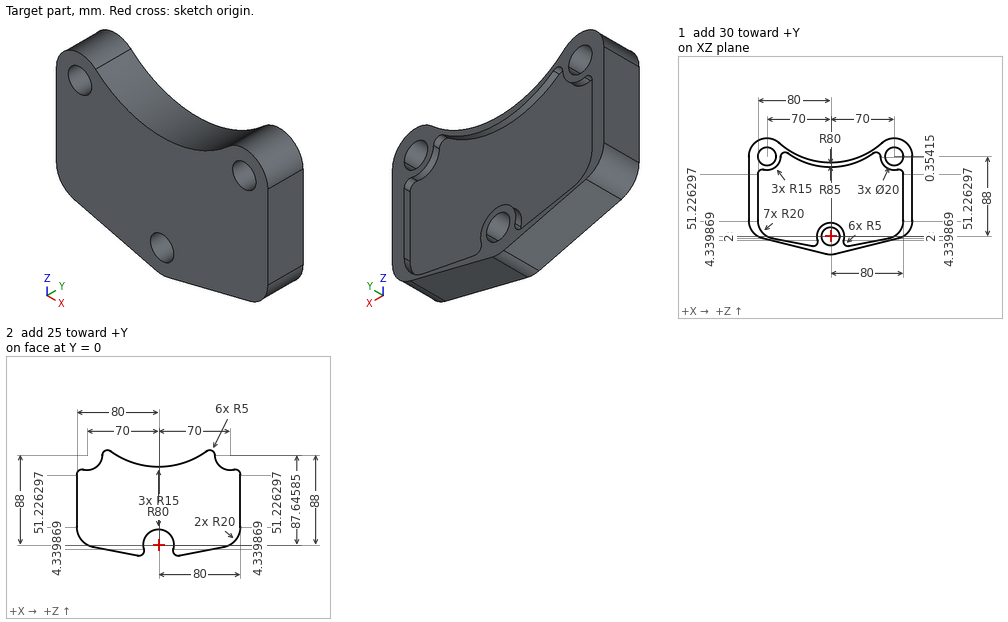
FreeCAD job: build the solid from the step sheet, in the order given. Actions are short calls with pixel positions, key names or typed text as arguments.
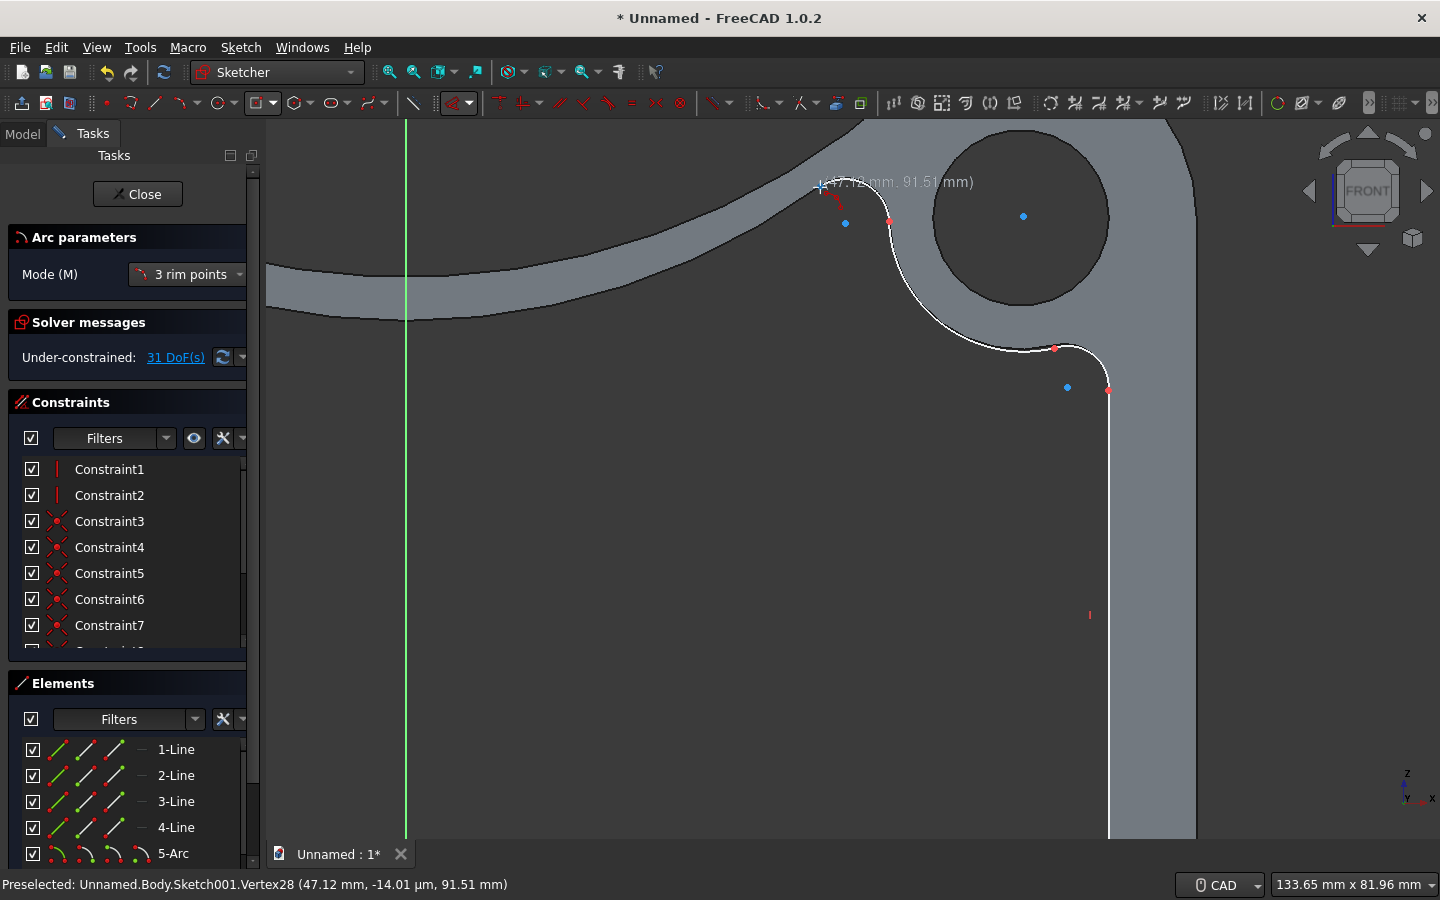
scroll(1093, 353, down, 4)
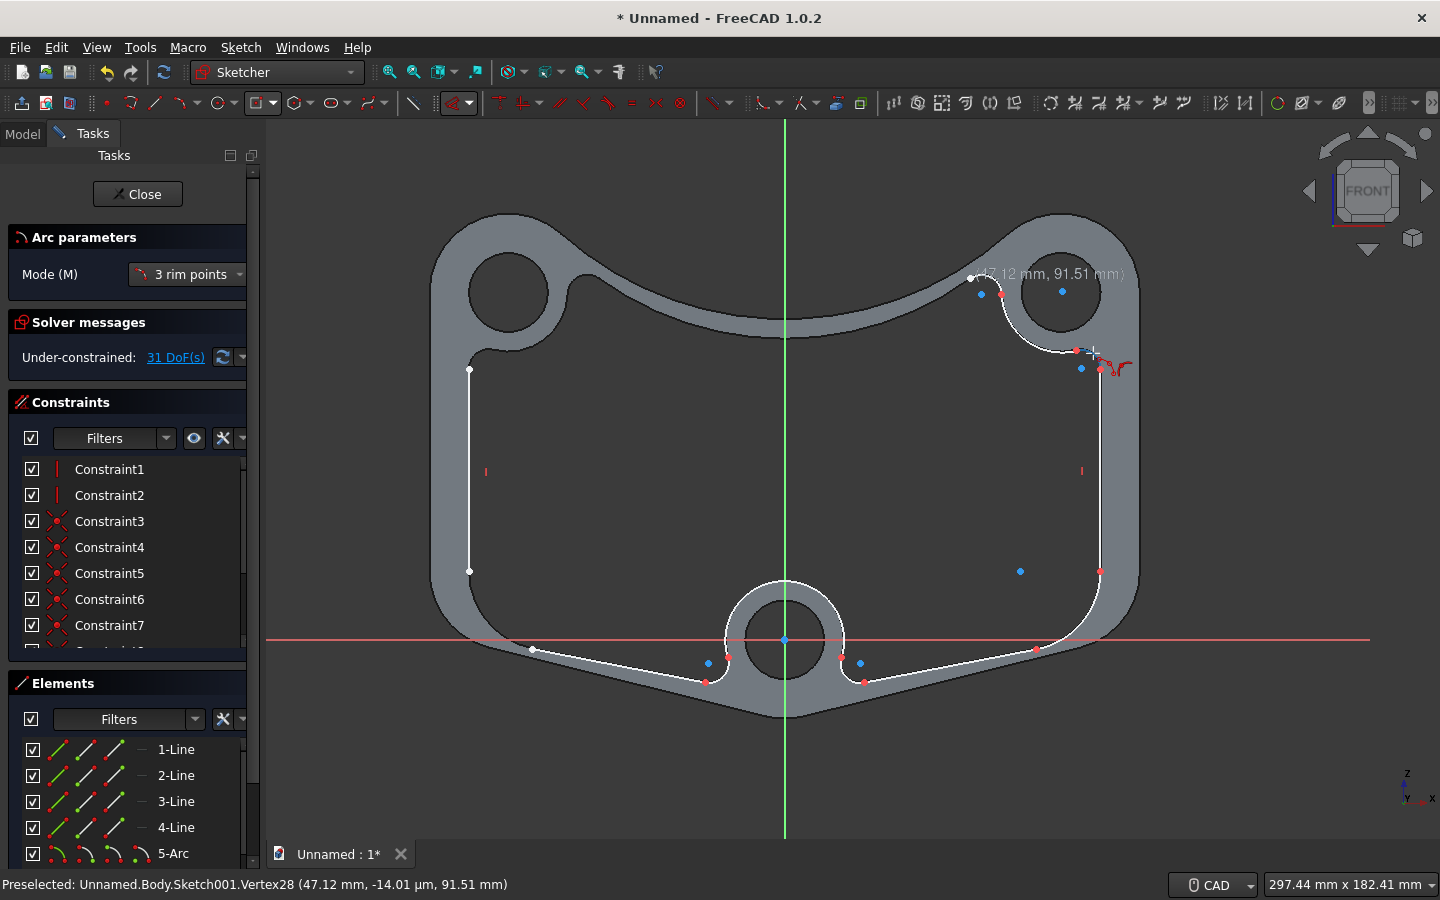
click(599, 278)
click(745, 336)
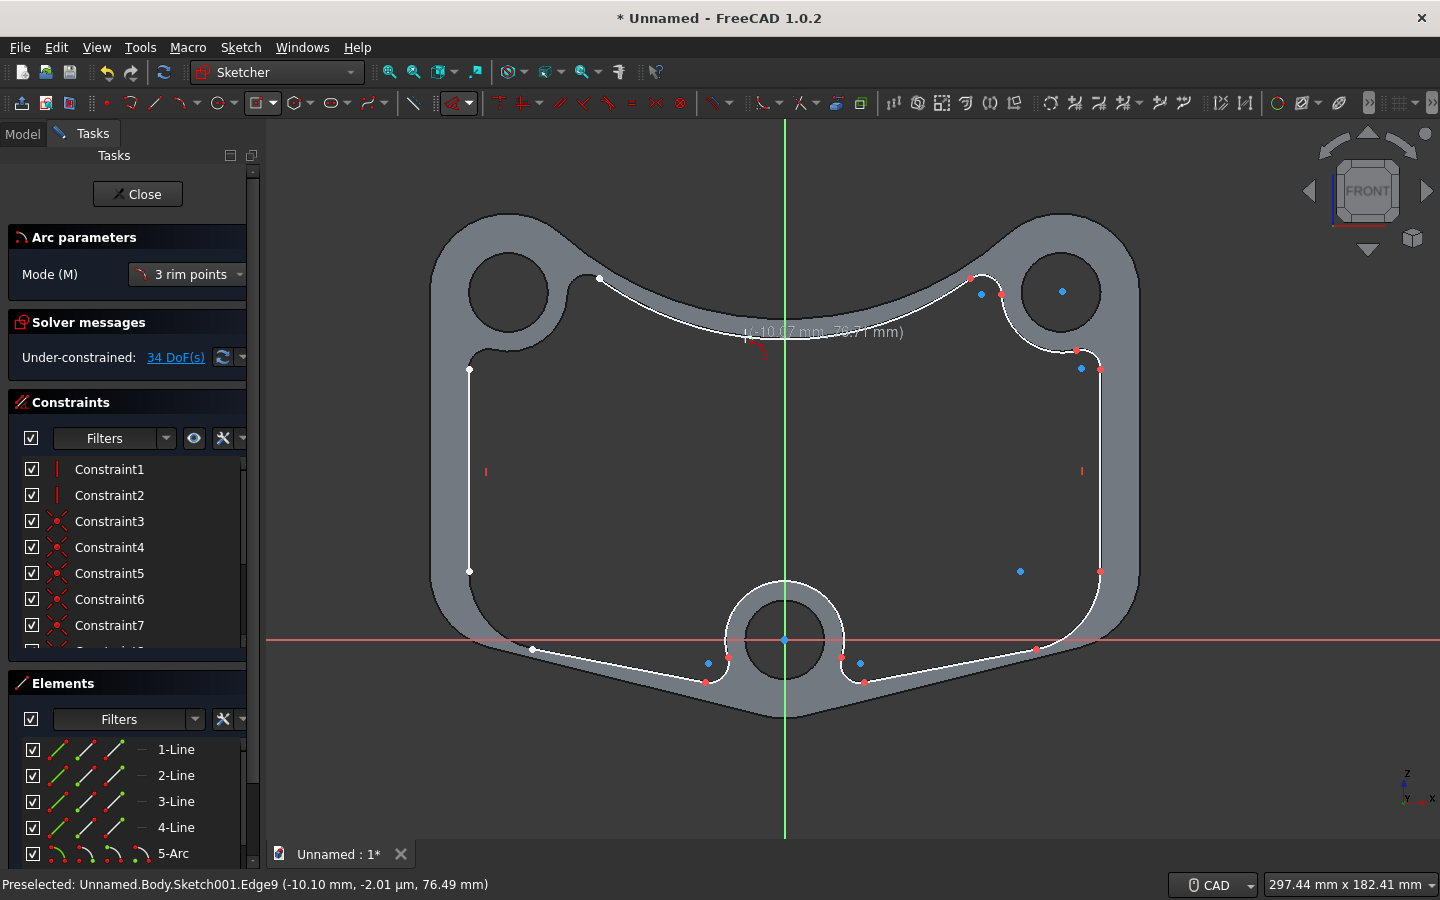
click(599, 279)
click(568, 294)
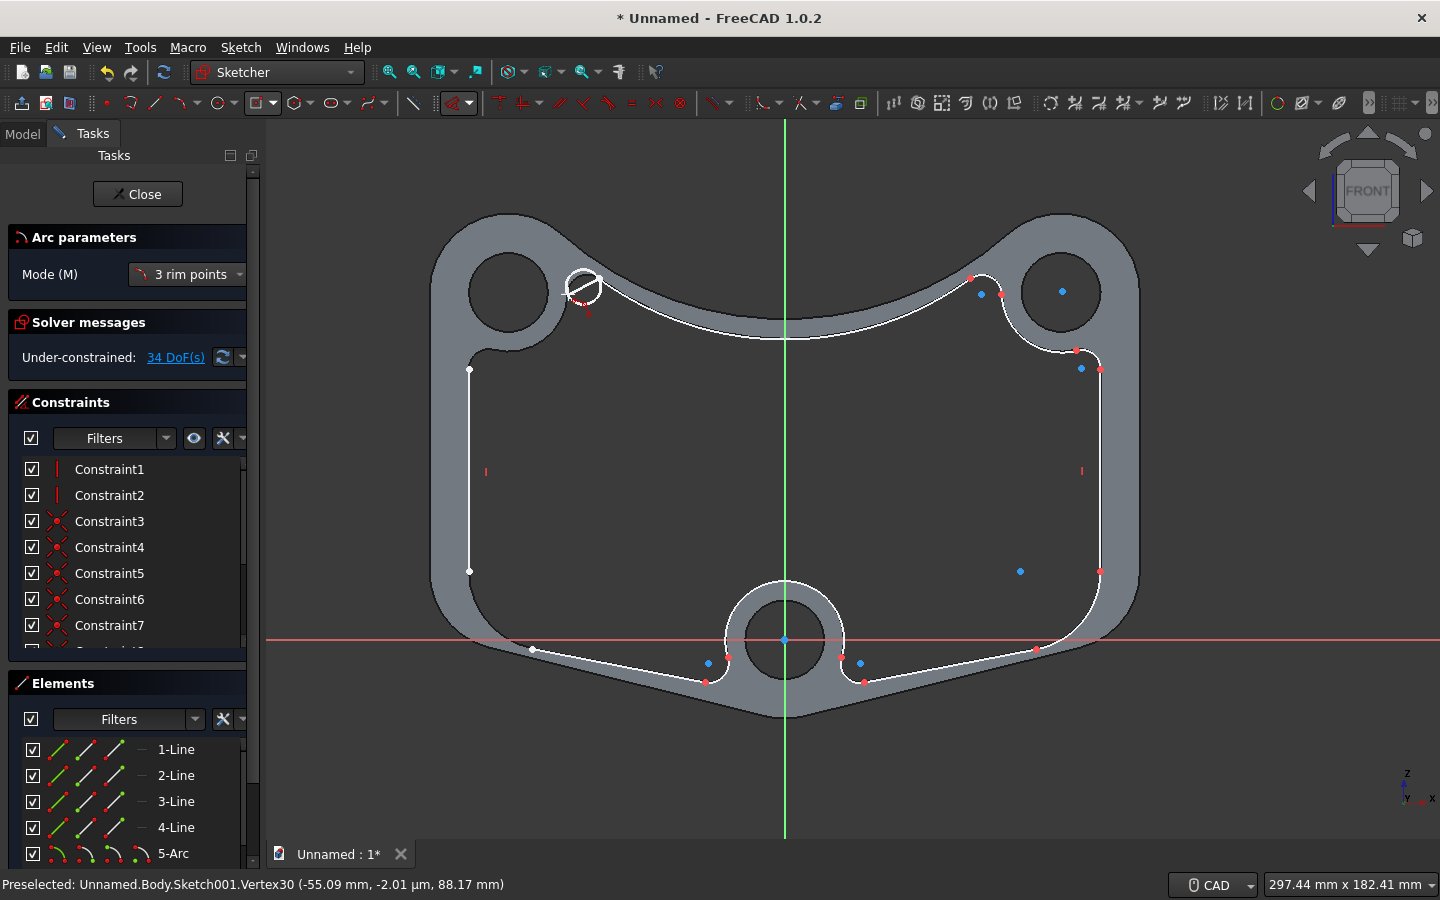
scroll(579, 277, up, 3)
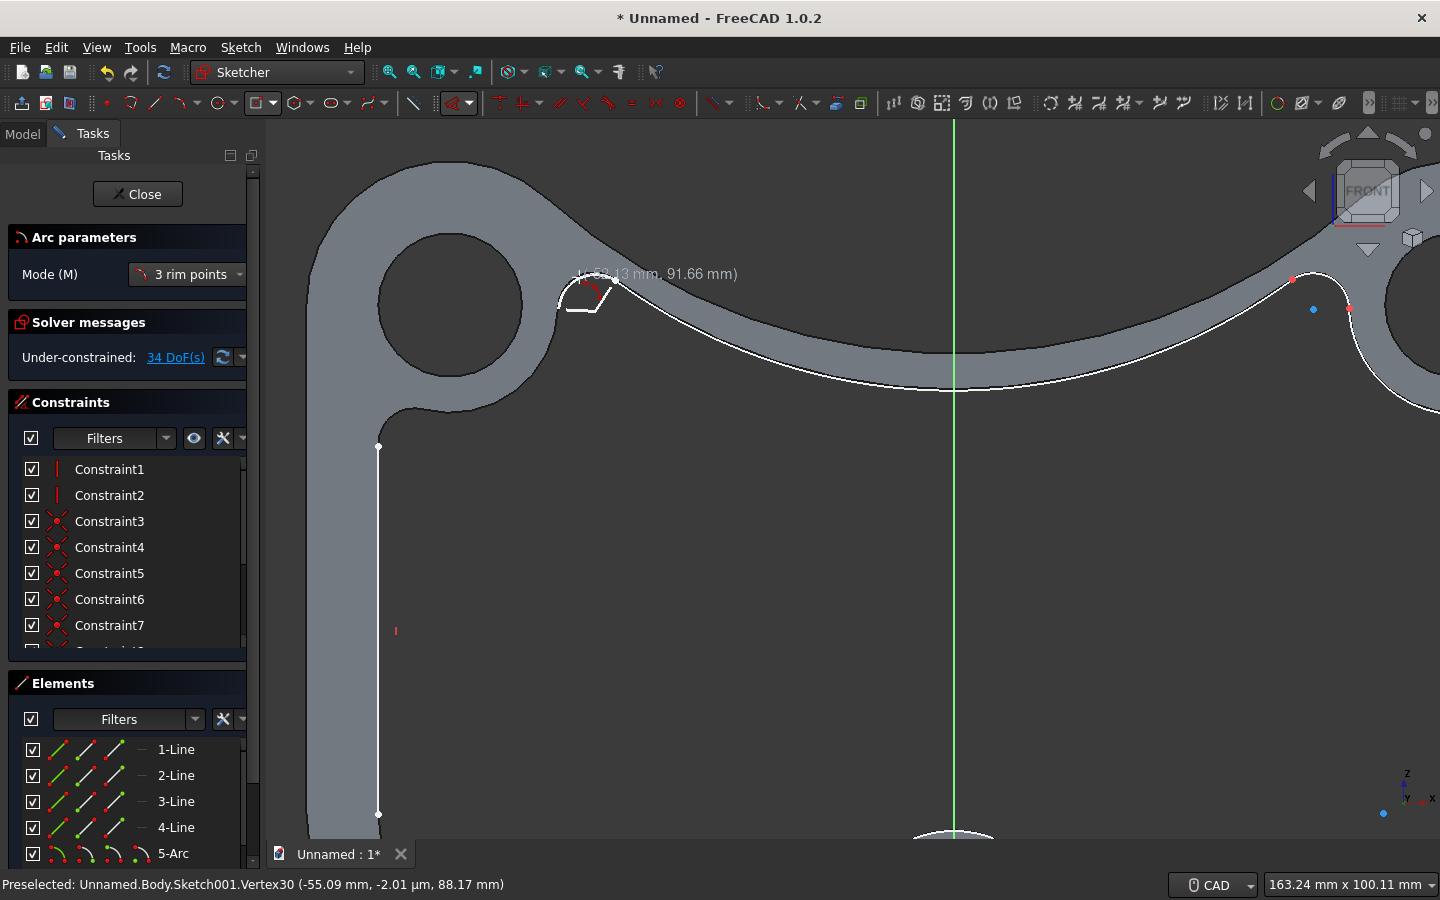
click(578, 276)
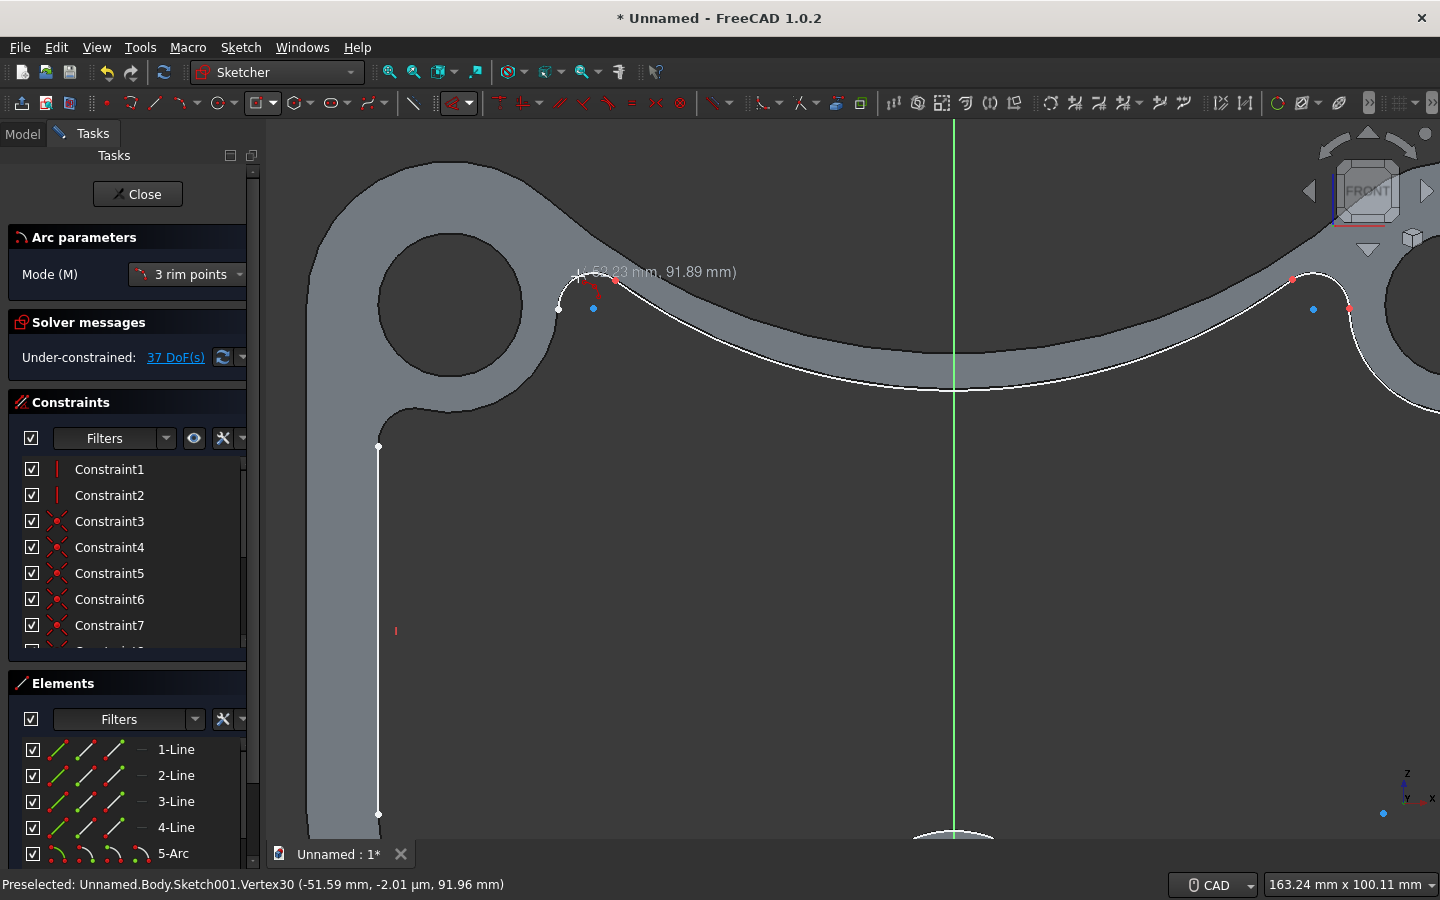
click(559, 310)
click(423, 409)
click(515, 391)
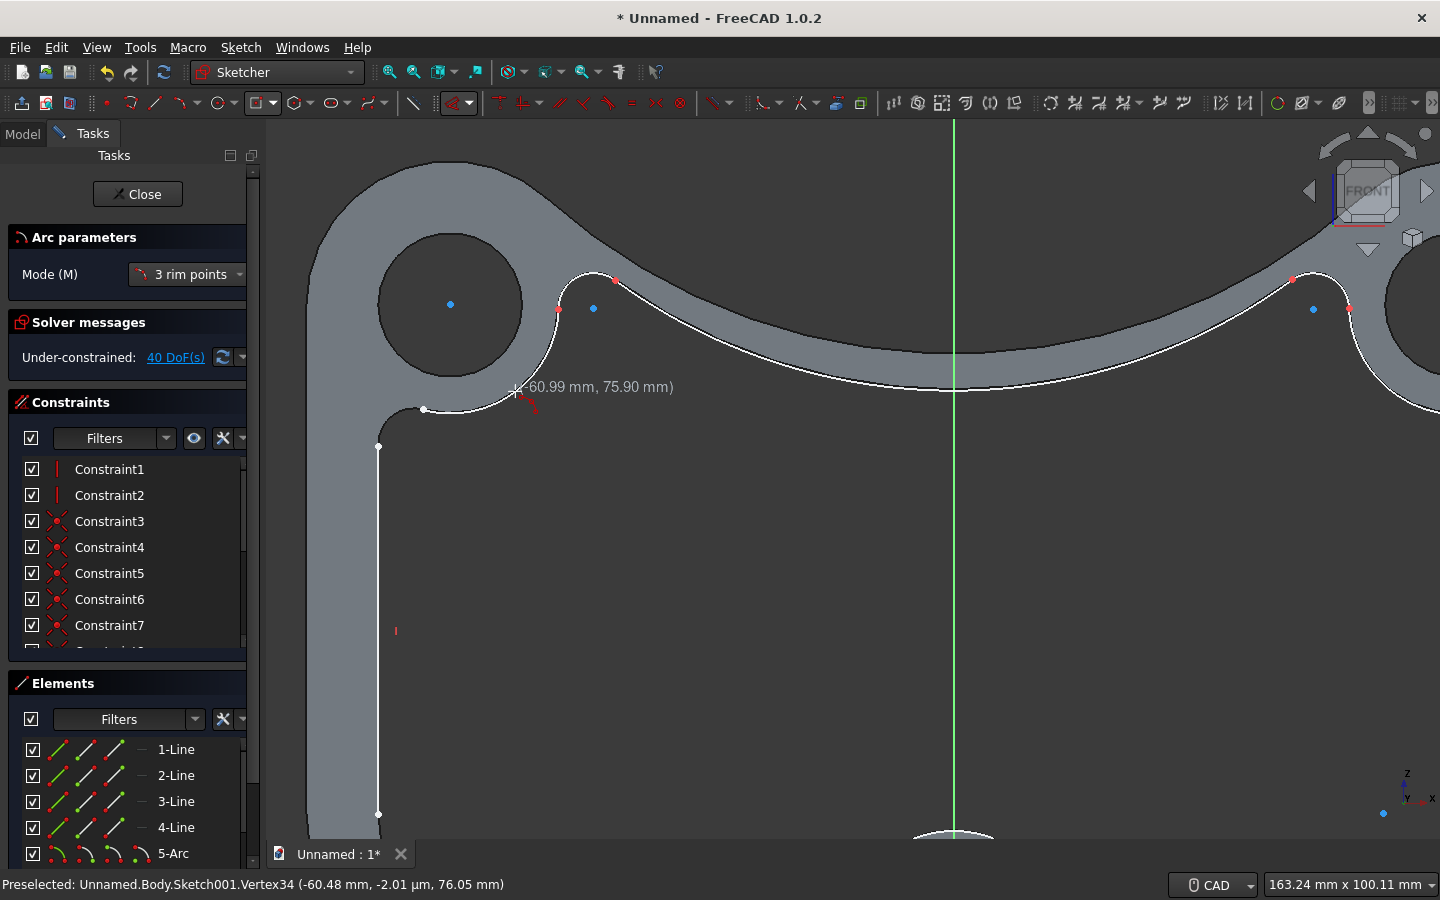
click(423, 410)
click(378, 446)
click(392, 416)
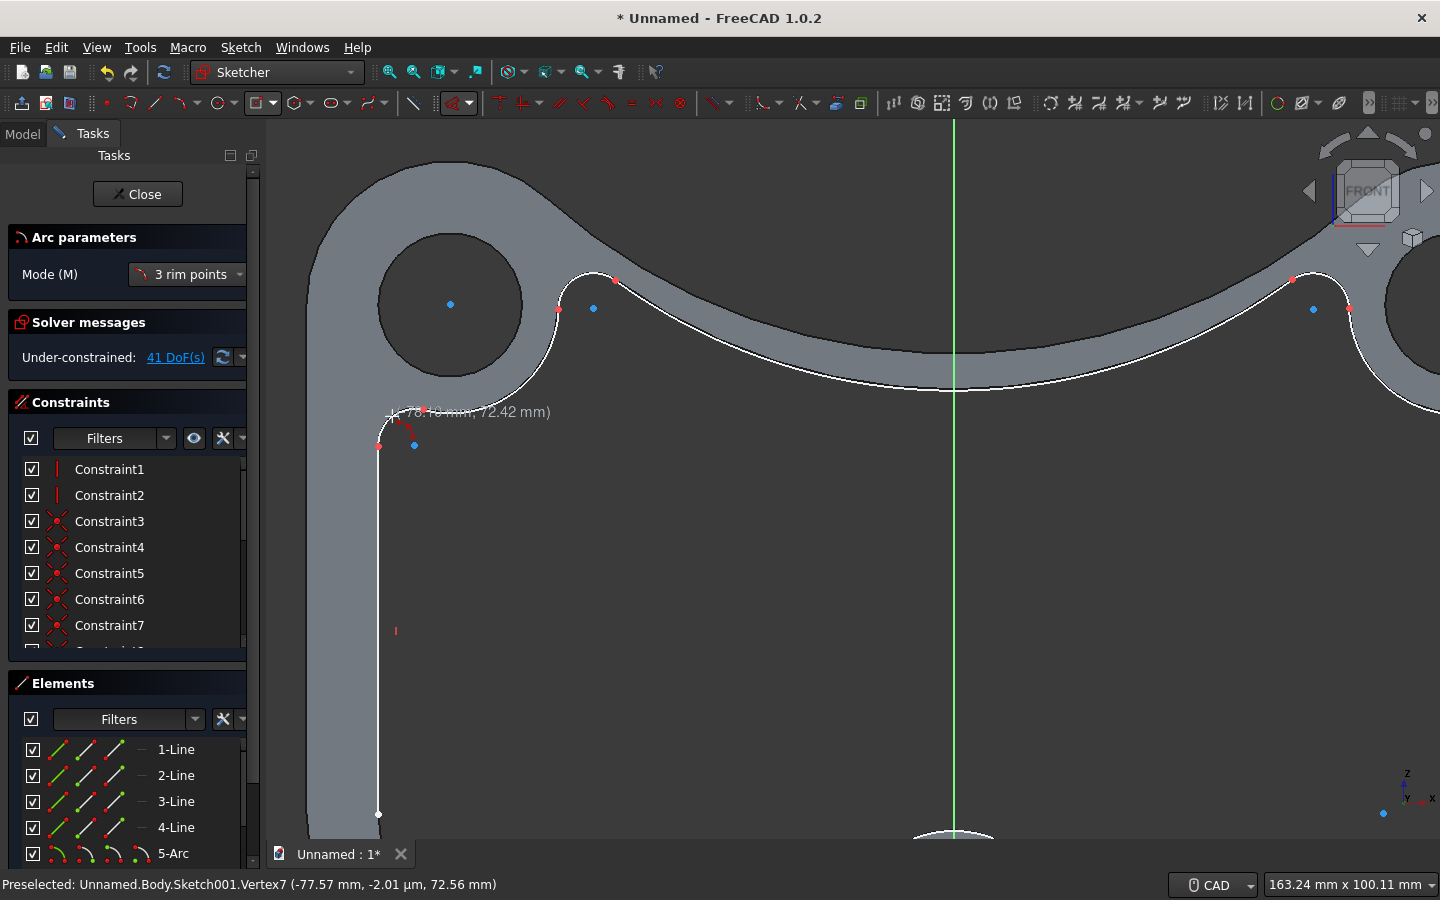
scroll(579, 277, down, 3)